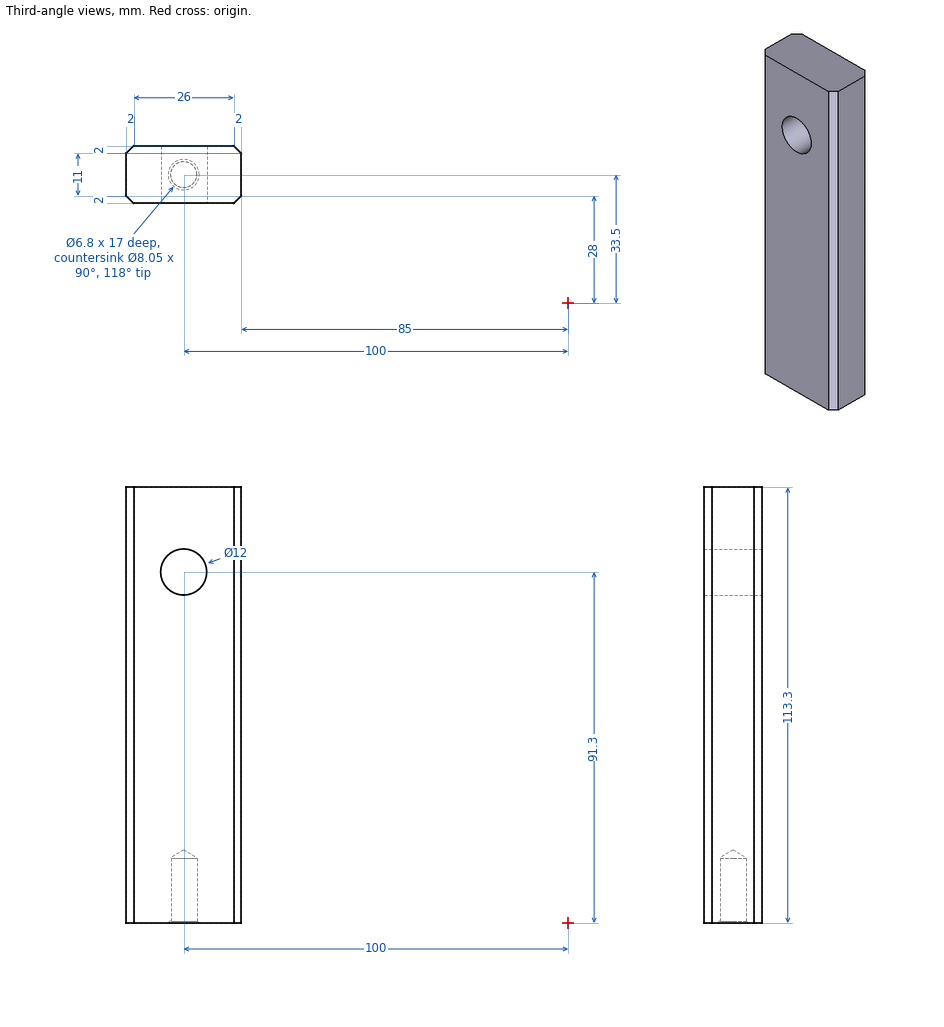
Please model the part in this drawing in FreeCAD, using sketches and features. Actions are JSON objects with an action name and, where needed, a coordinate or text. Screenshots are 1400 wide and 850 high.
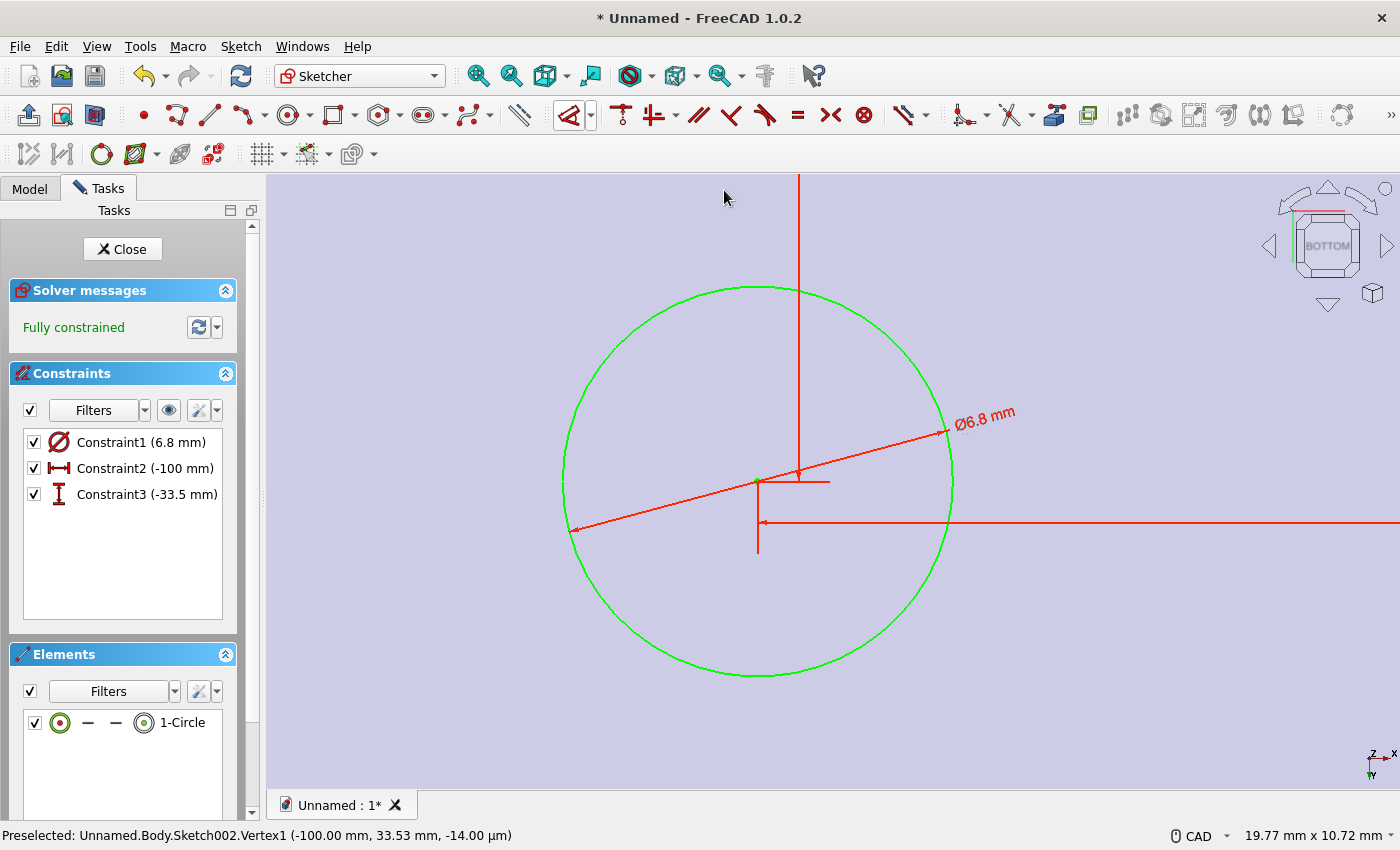
{"action": "left_click", "coordinate": [123, 249]}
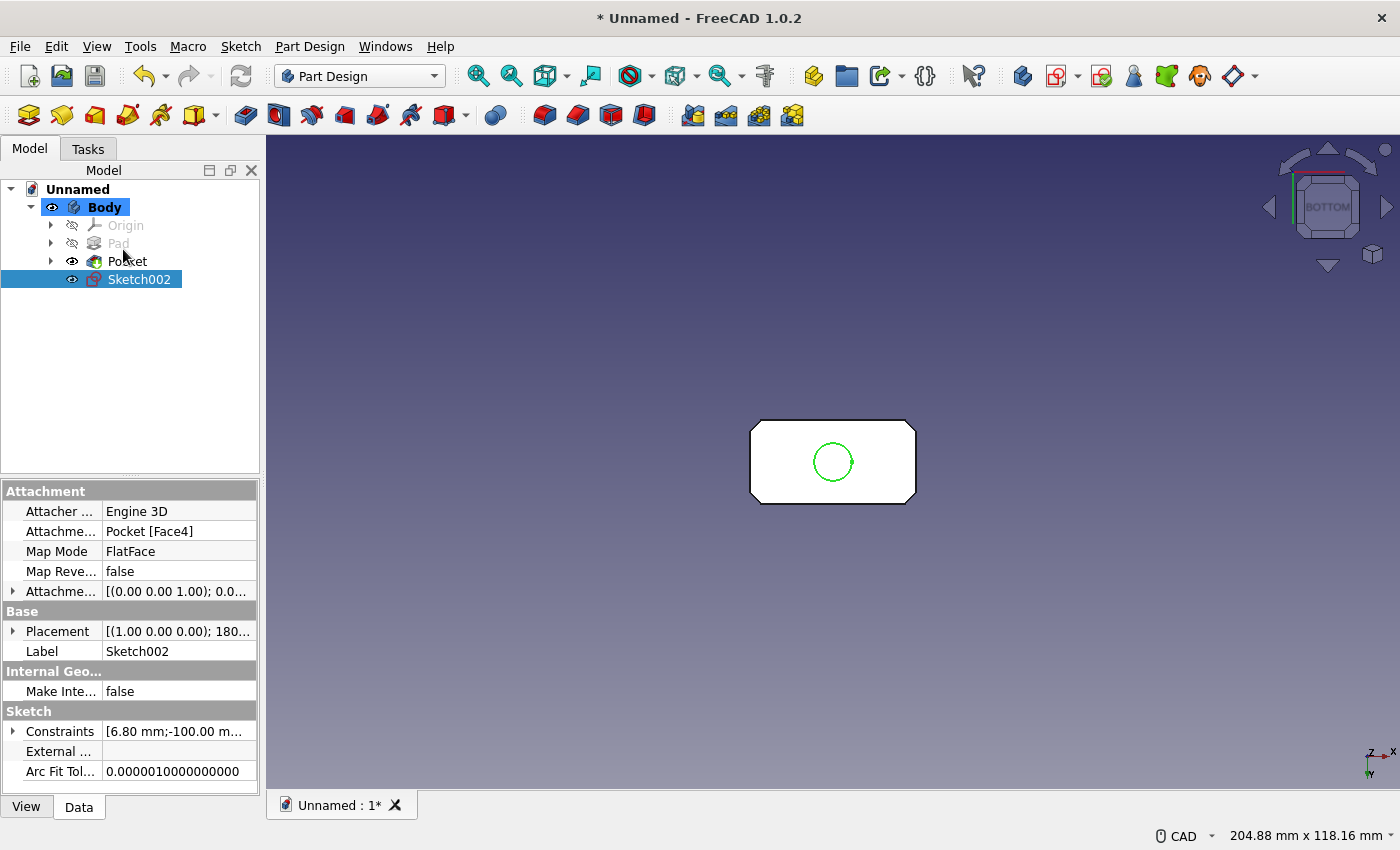
{"action": "left_click", "coordinate": [279, 116]}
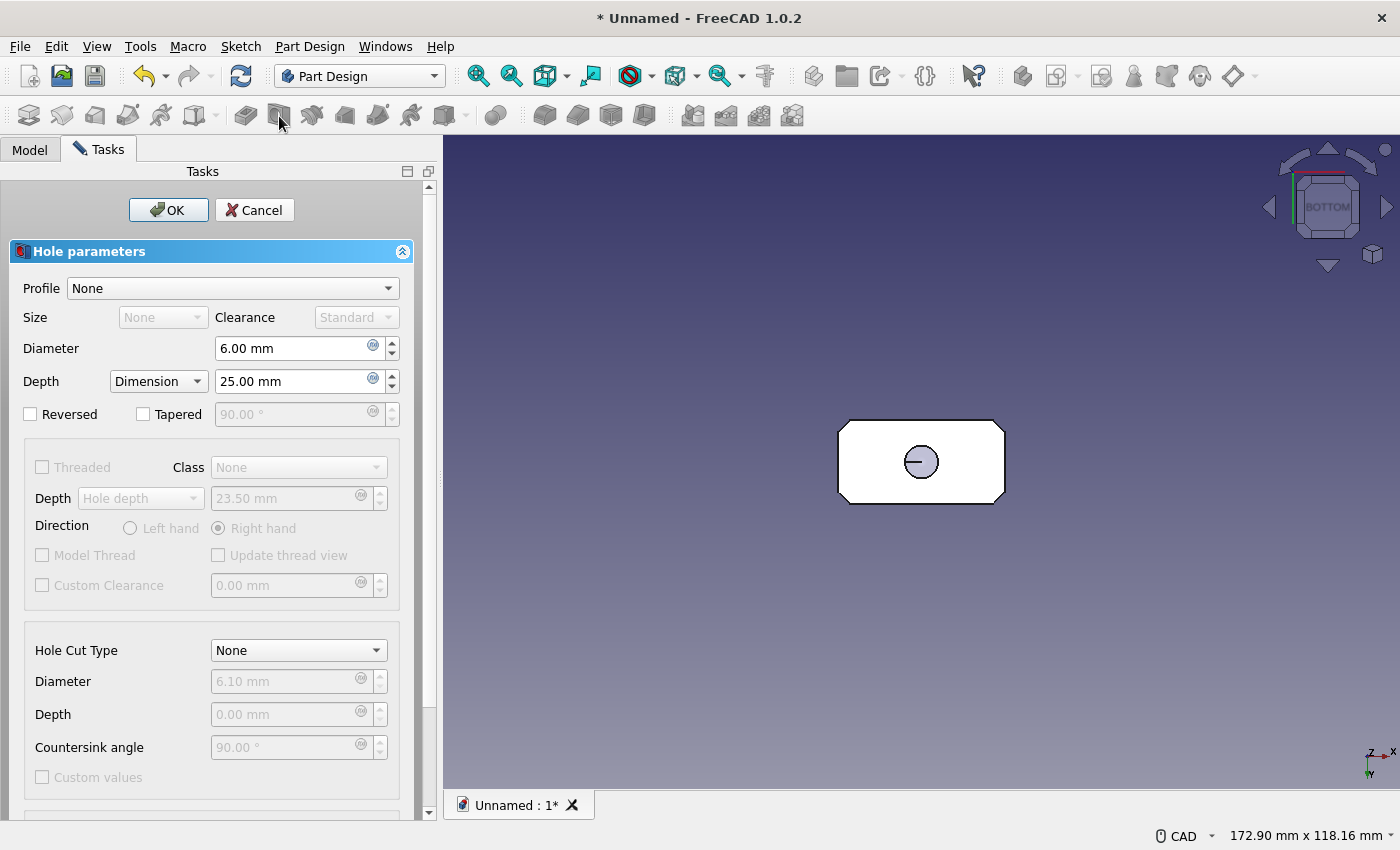
{"action": "triple_click", "coordinate": [300, 348]}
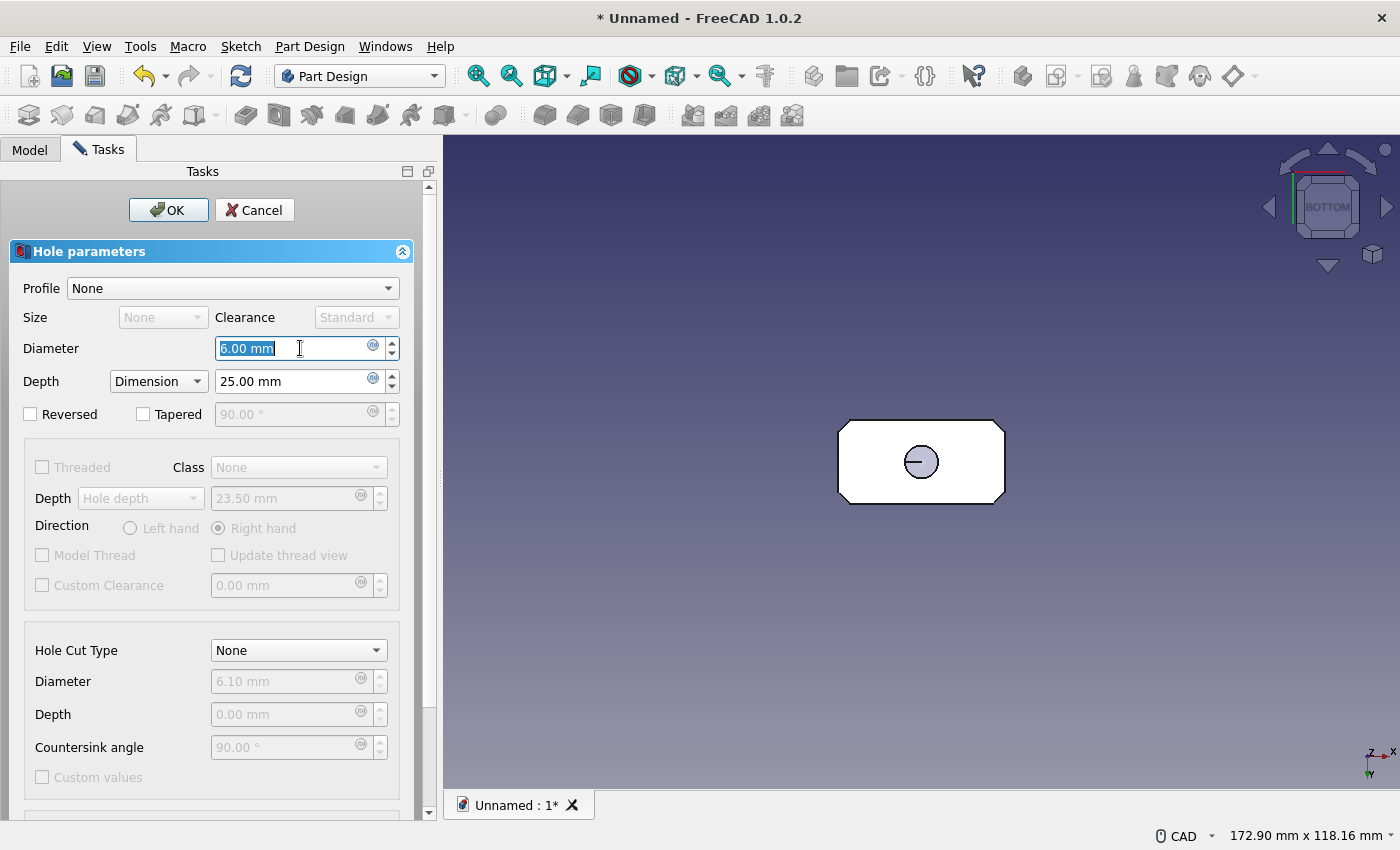
{"action": "type", "text": "6.8"}
{"action": "key", "text": "Tab"}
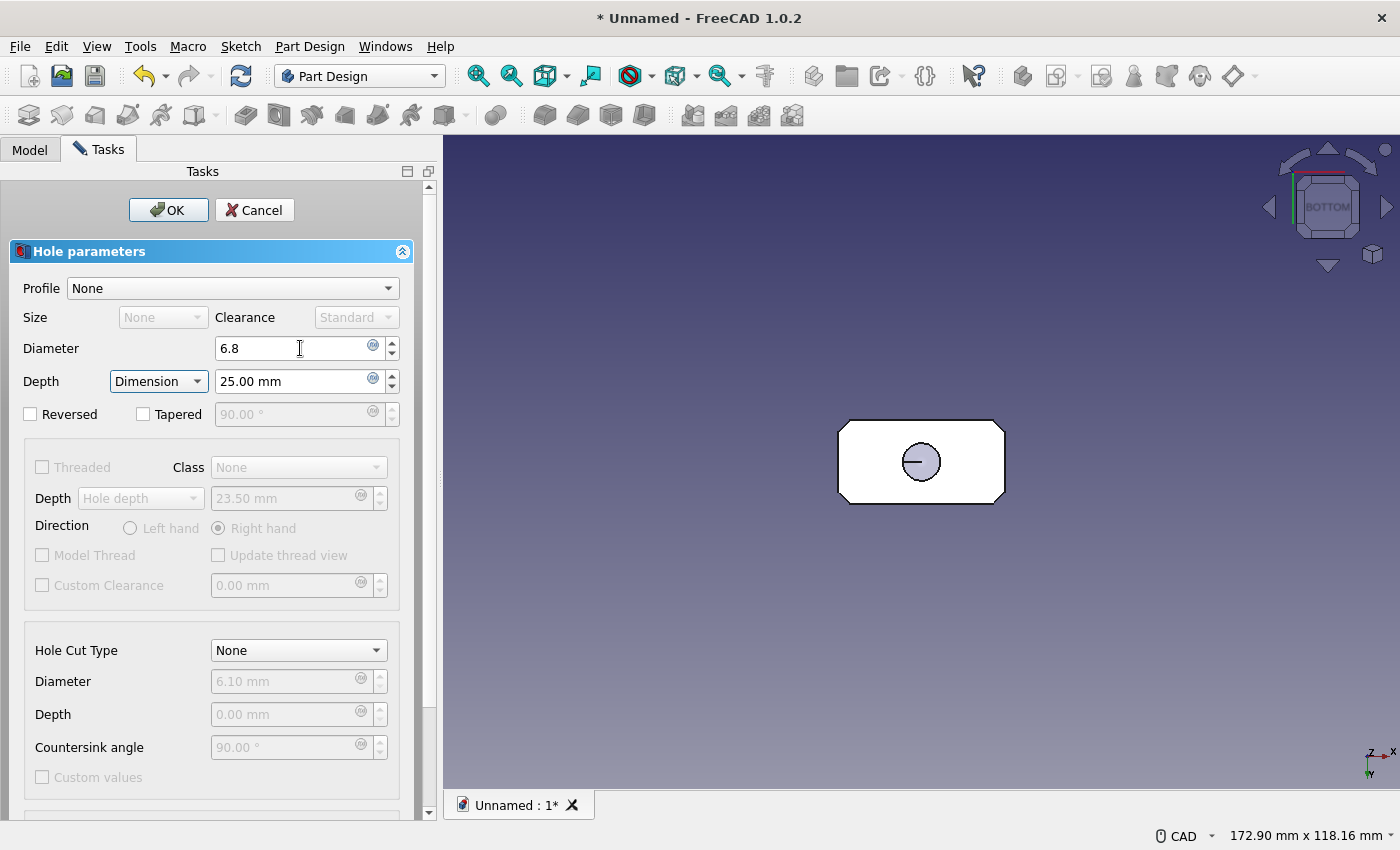
{"action": "triple_click", "coordinate": [300, 382]}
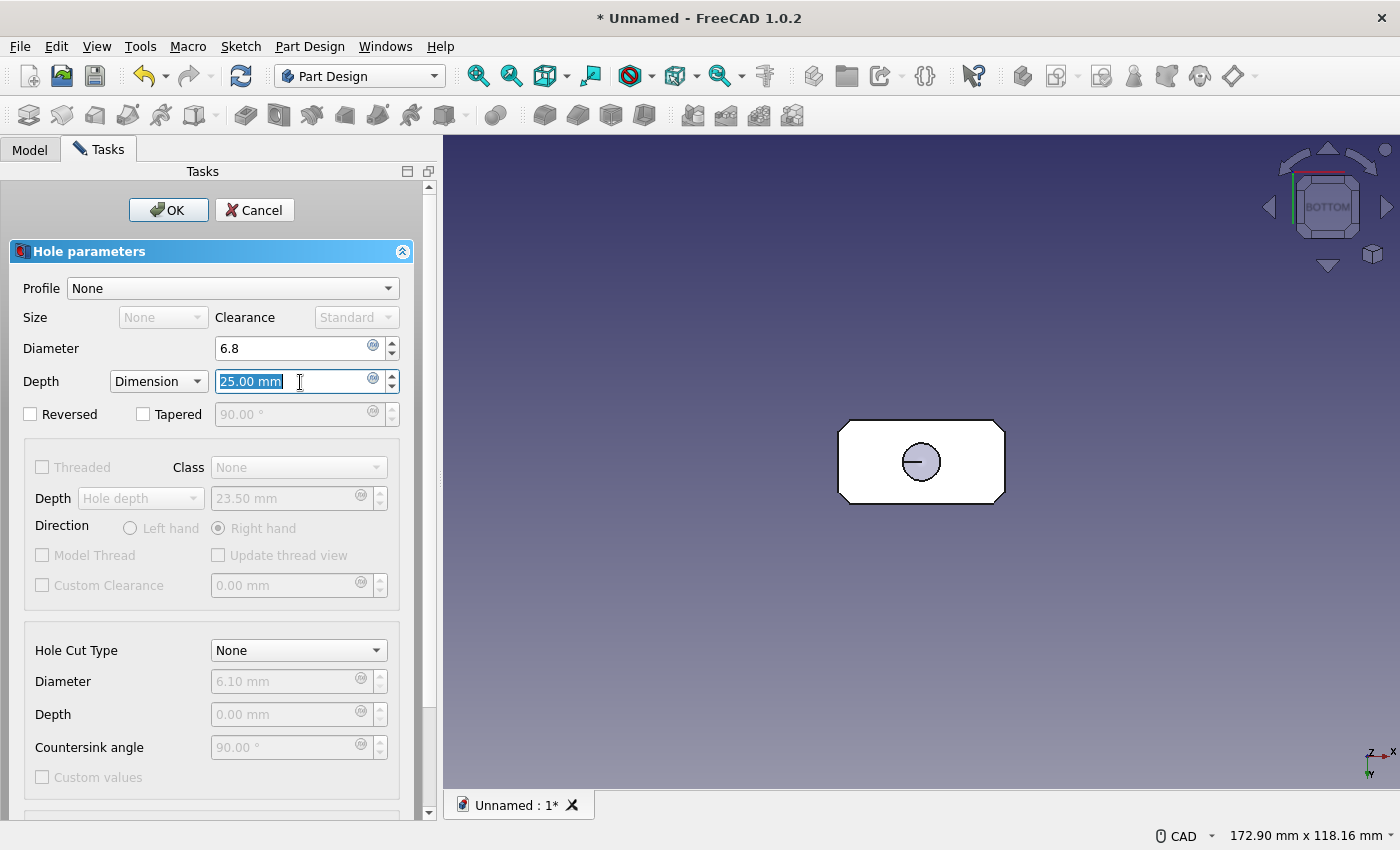
{"action": "type", "text": "17"}
{"action": "key", "text": "Tab"}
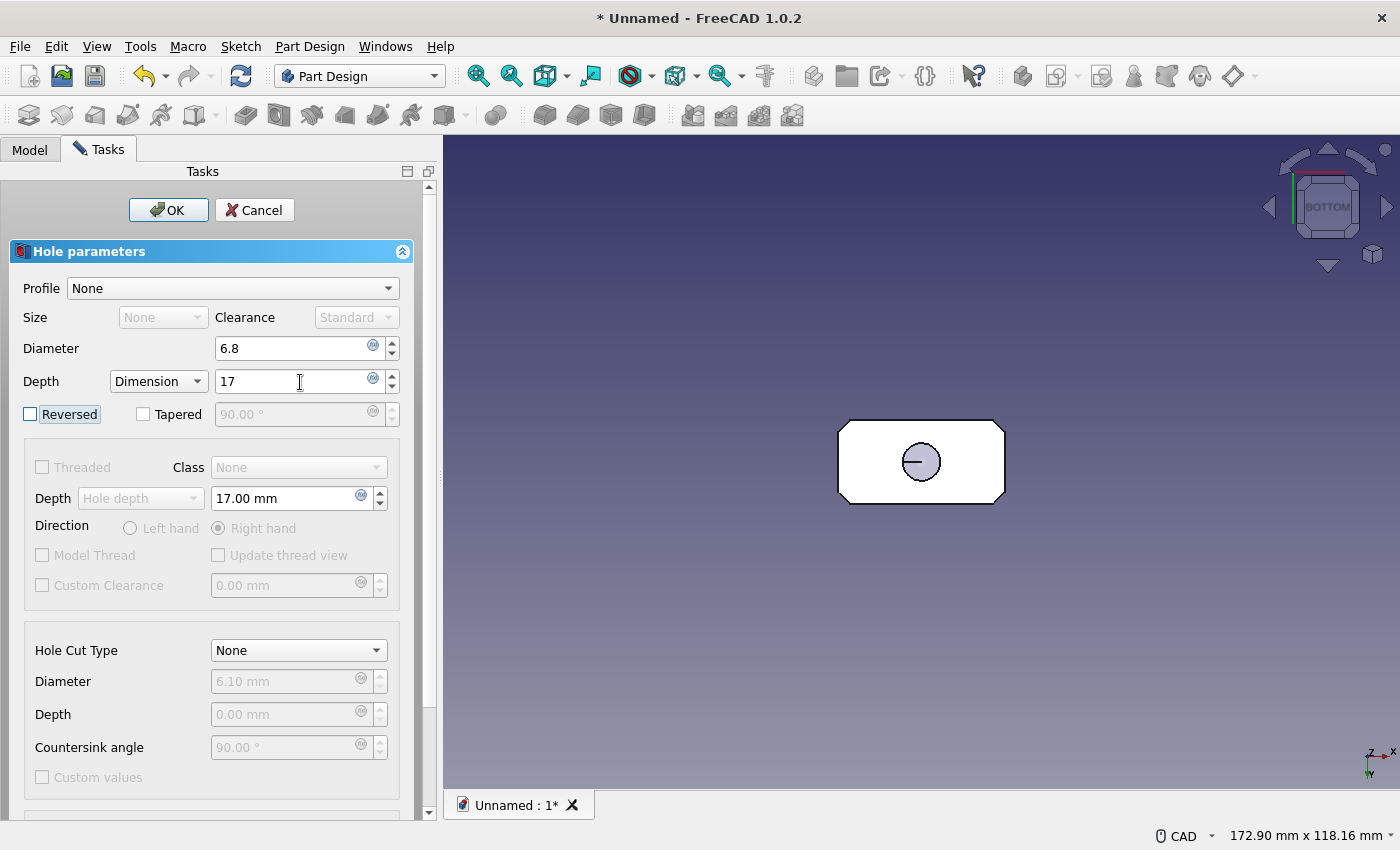
{"action": "left_click", "coordinate": [300, 650]}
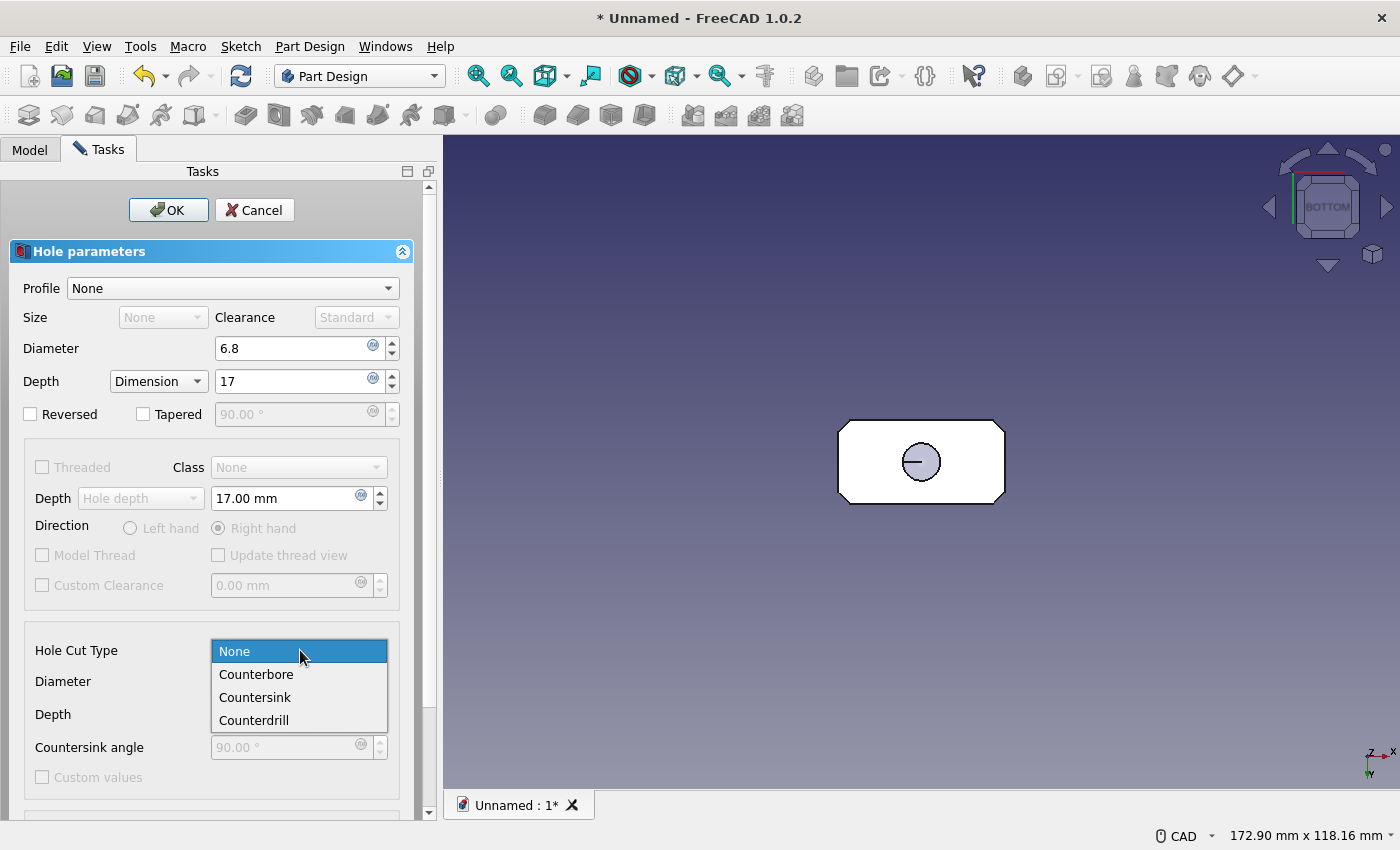
{"action": "left_click", "coordinate": [298, 698]}